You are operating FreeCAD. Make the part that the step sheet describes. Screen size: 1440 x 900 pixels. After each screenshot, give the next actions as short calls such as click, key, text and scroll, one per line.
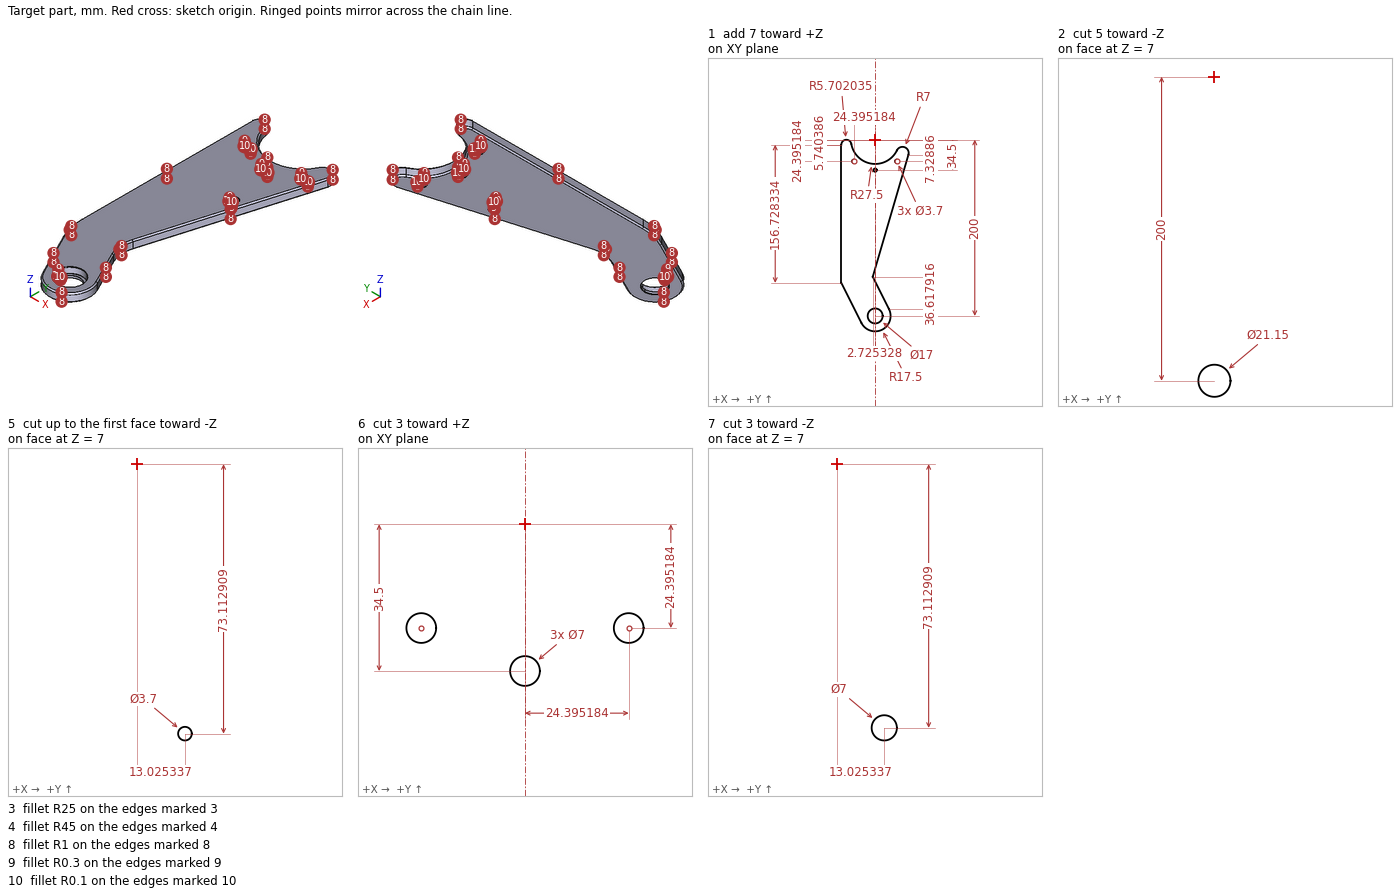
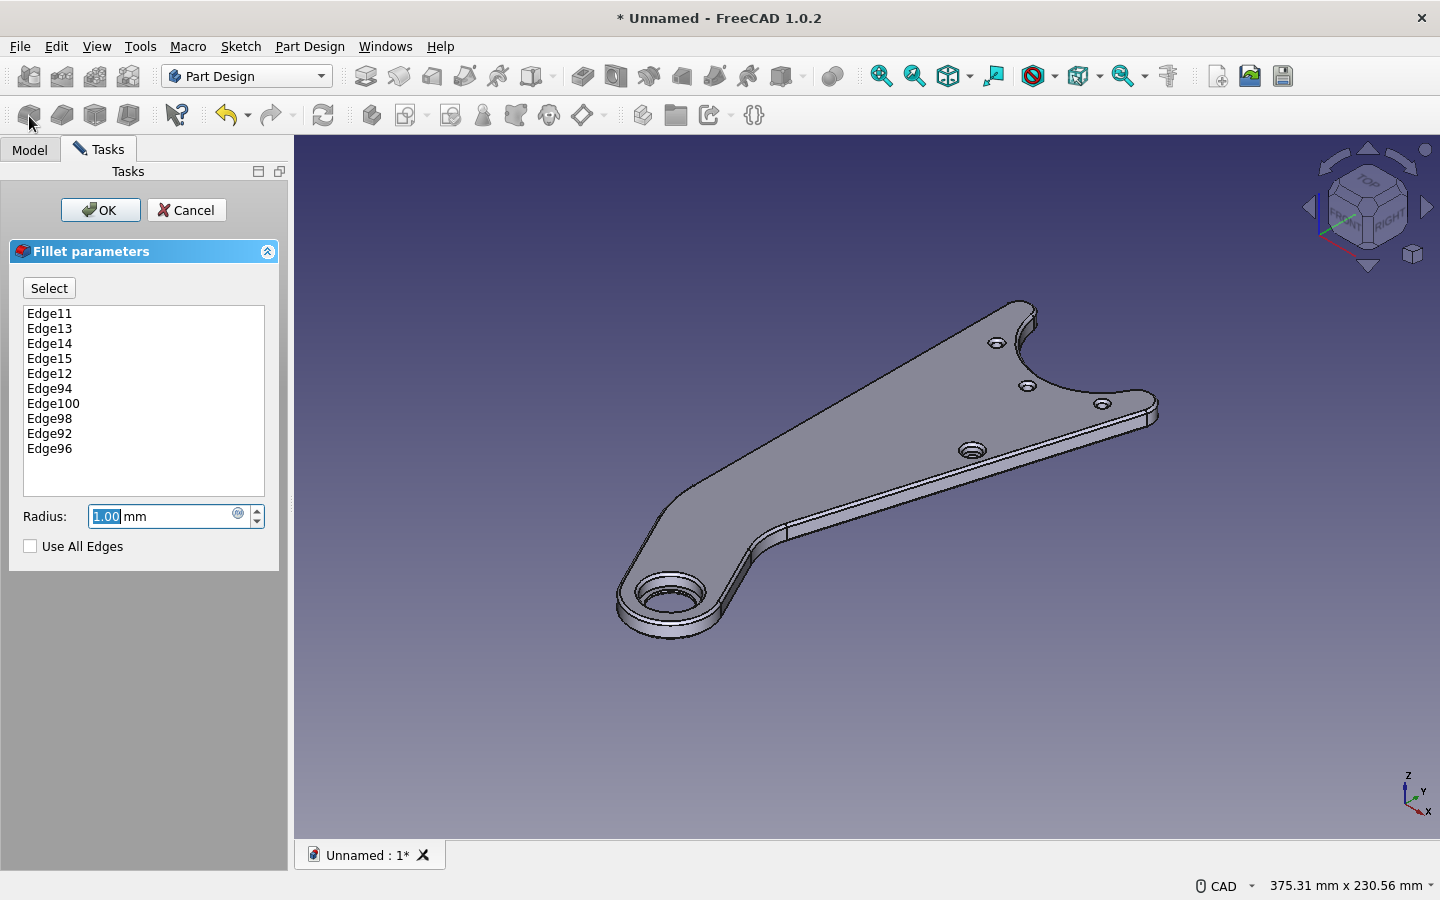
text(0.3)
key(Tab)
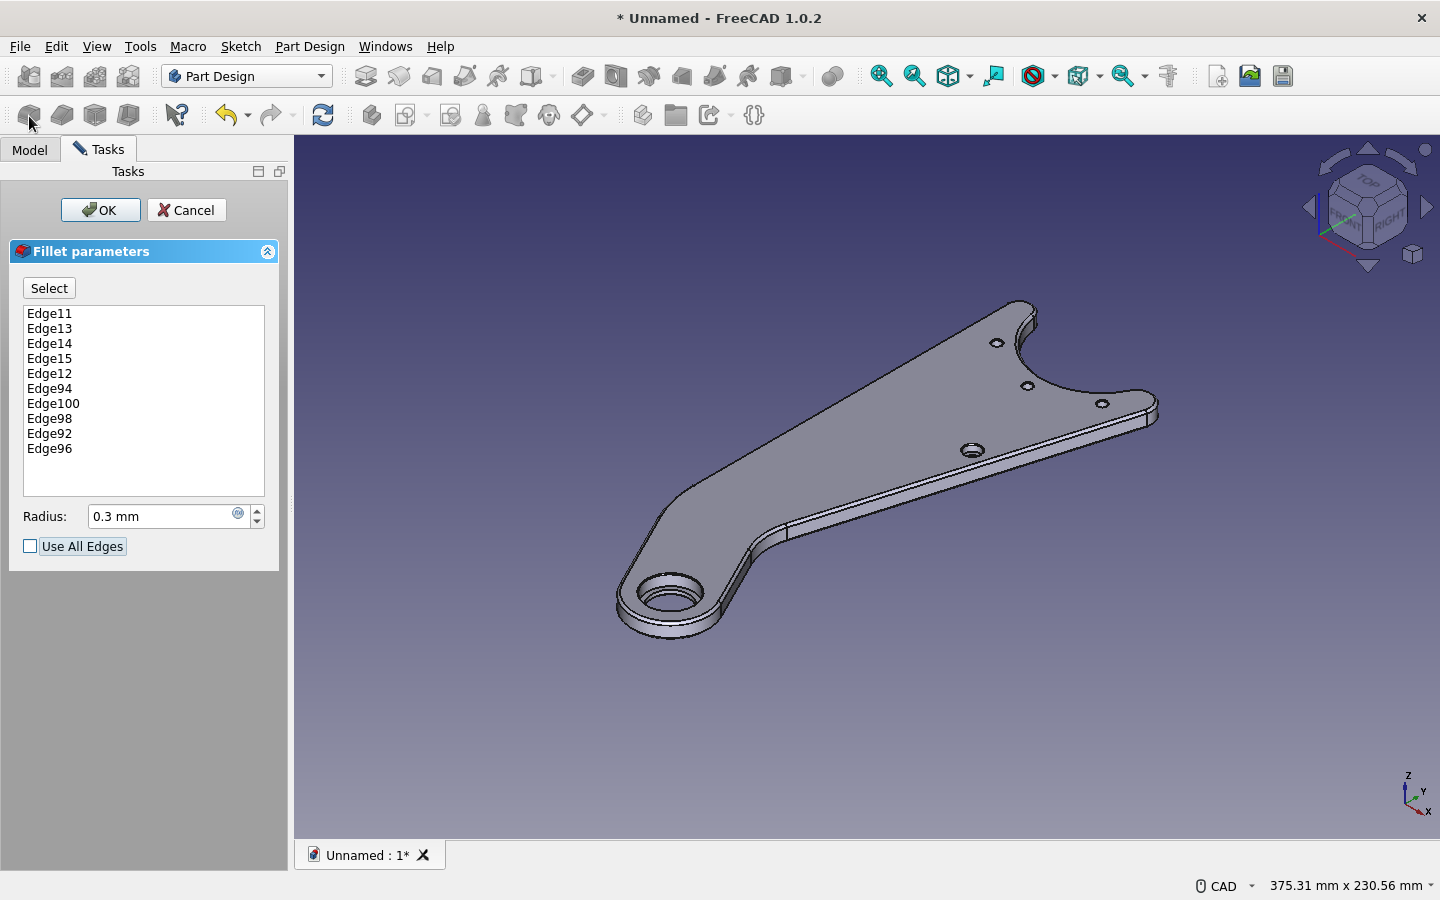
click(101, 210)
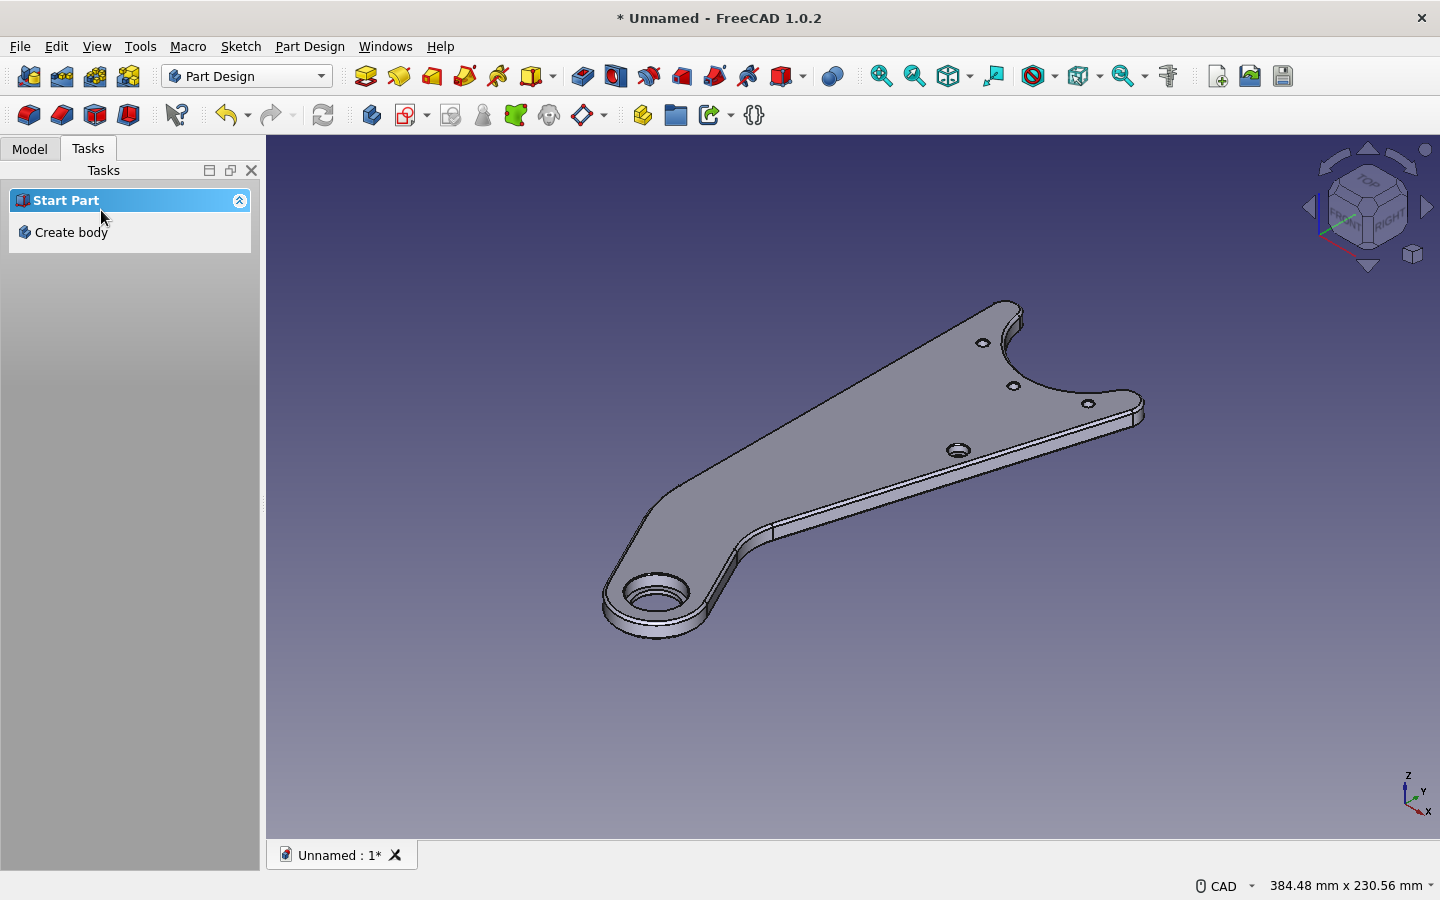
click(638, 593)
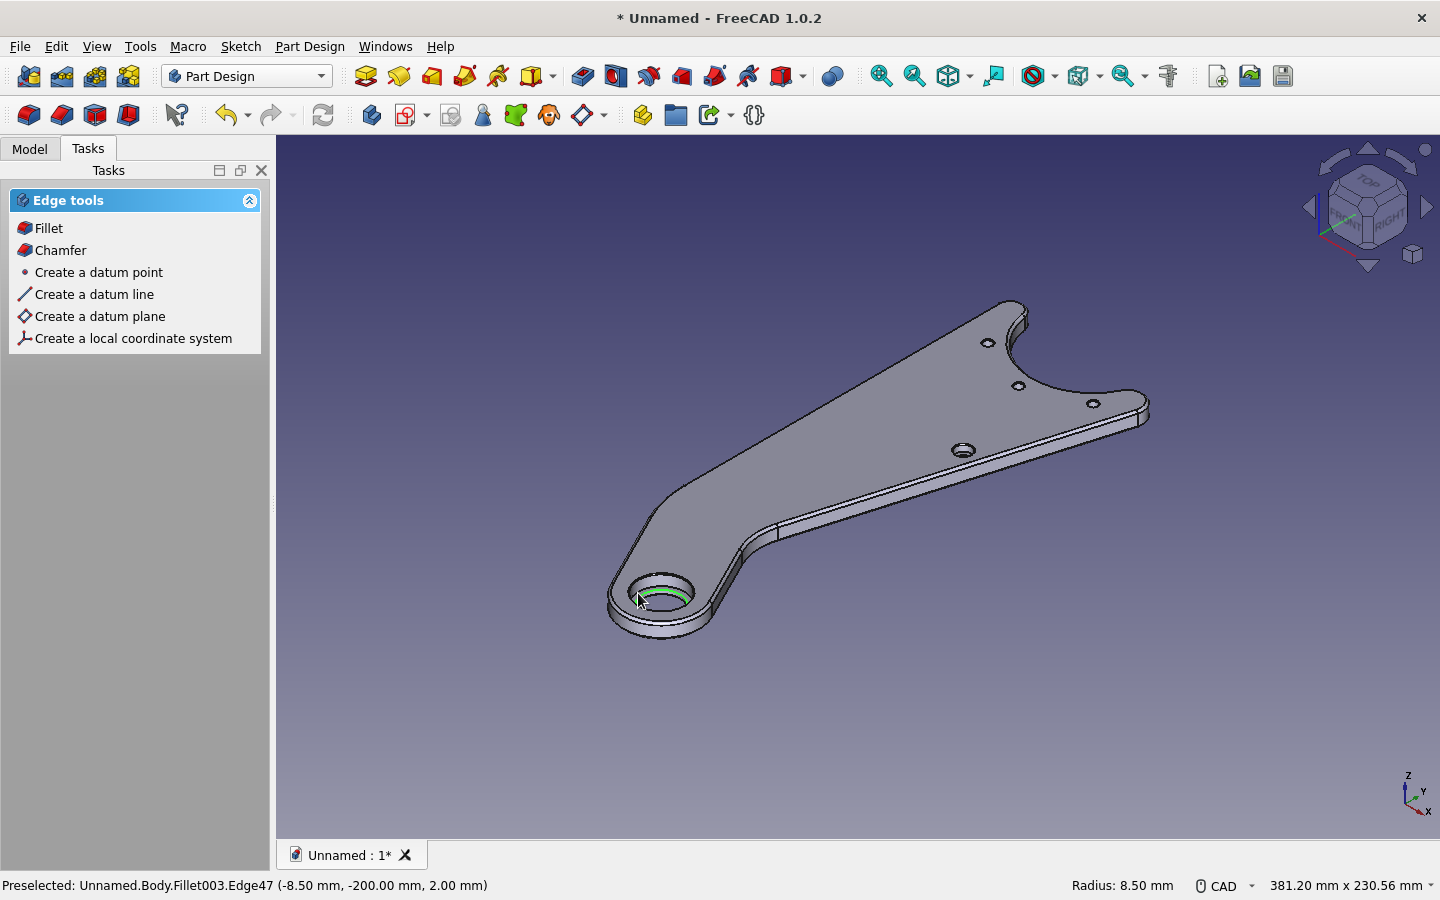
key(2)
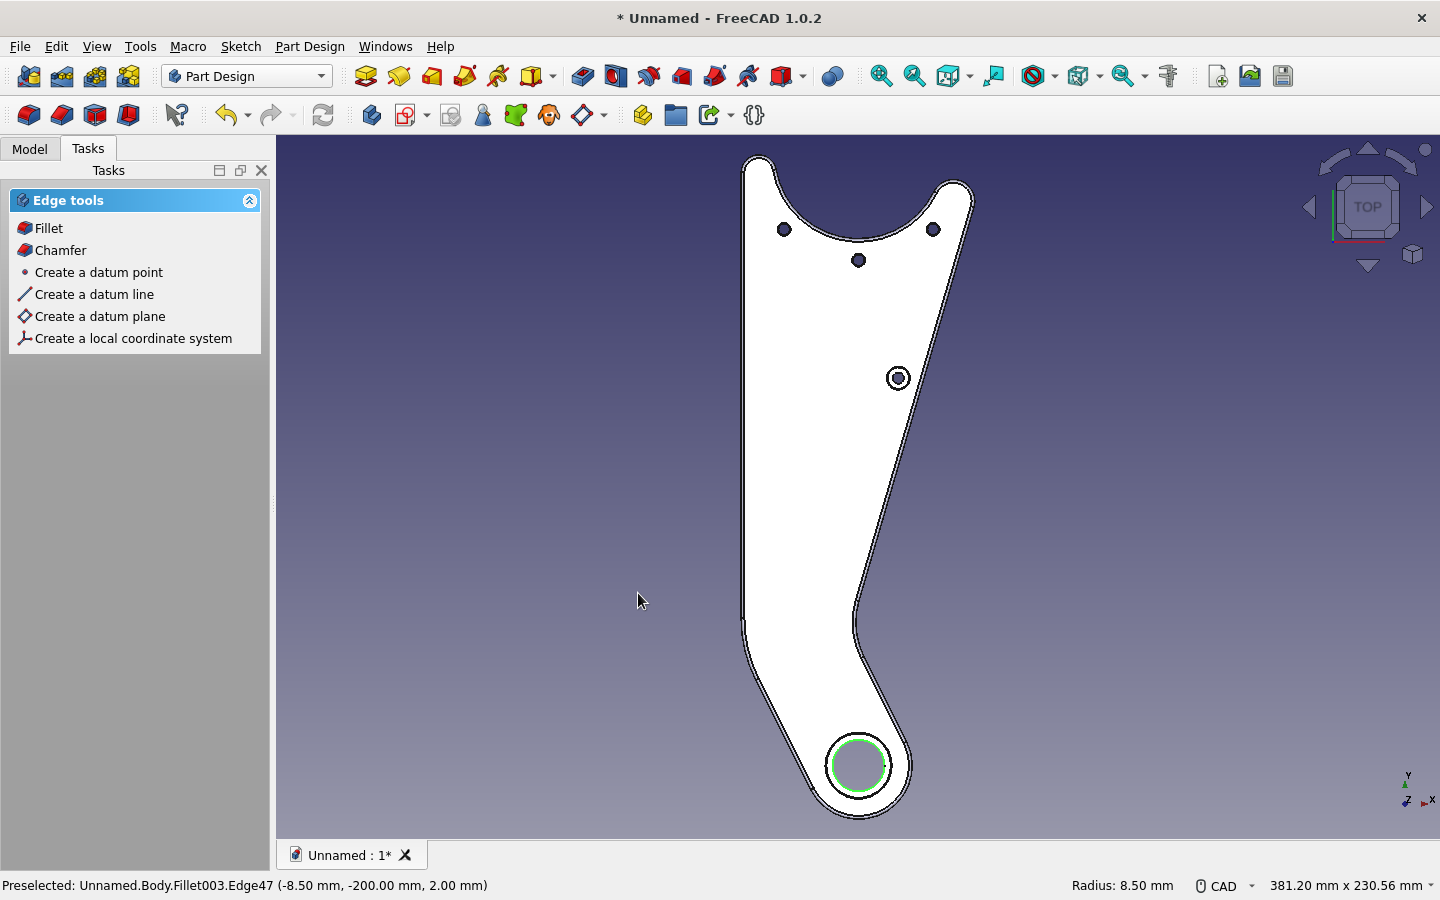
key(0)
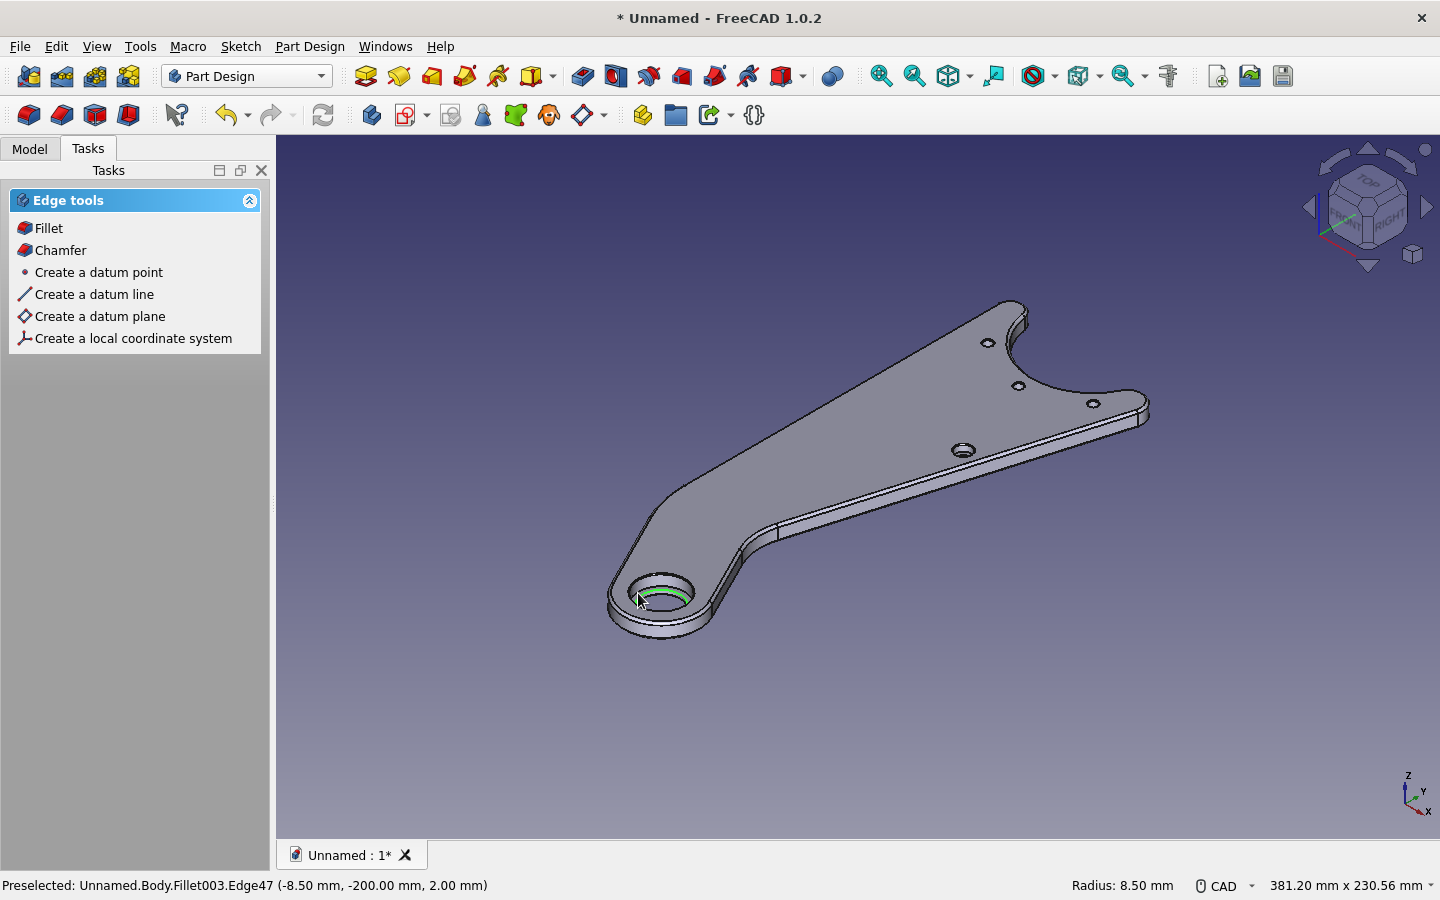
key(1)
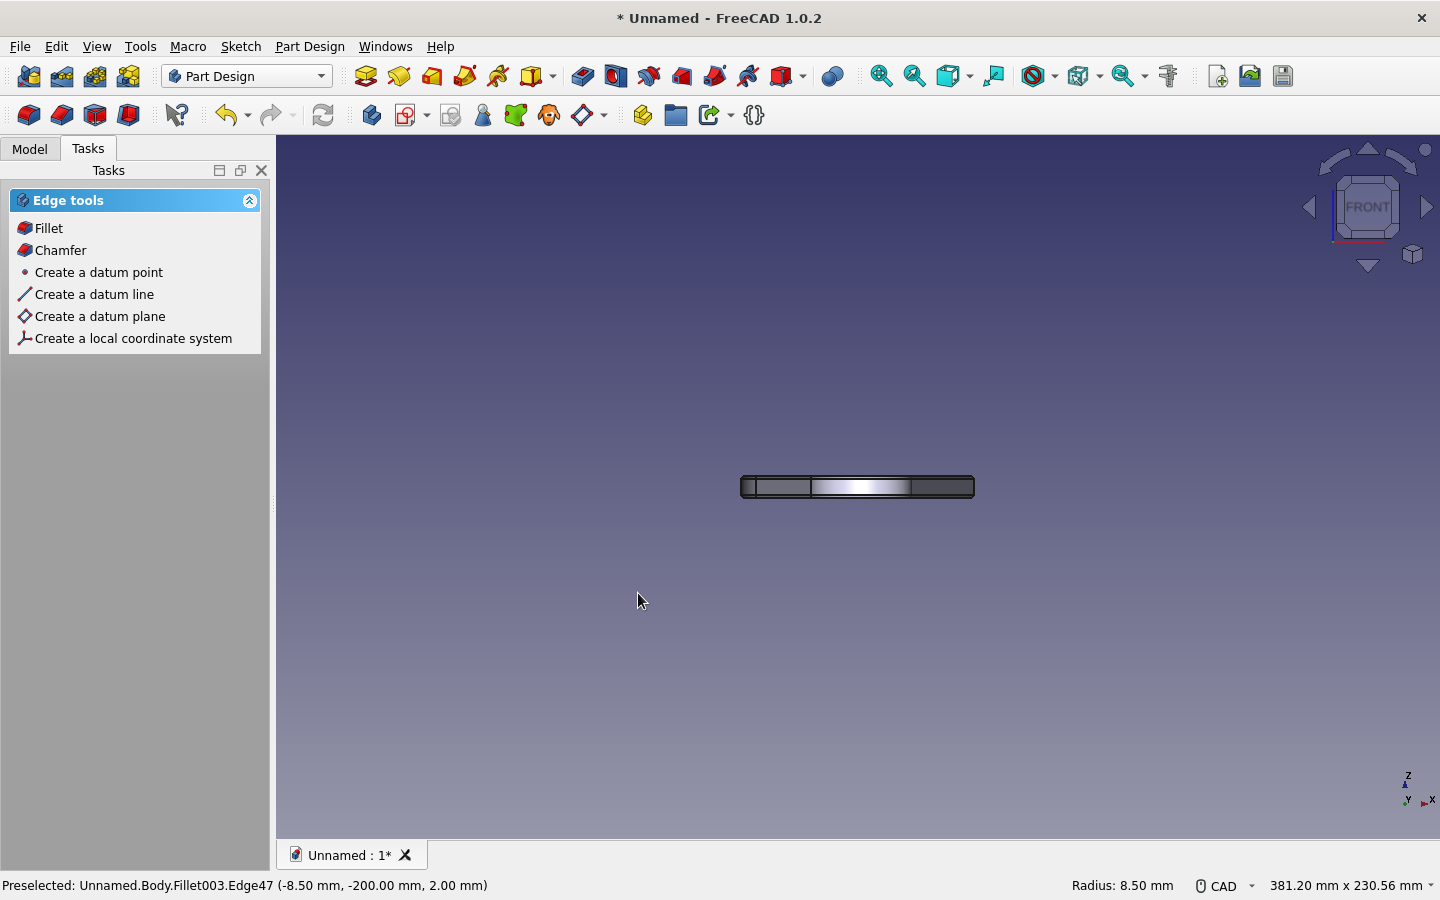
click(882, 76)